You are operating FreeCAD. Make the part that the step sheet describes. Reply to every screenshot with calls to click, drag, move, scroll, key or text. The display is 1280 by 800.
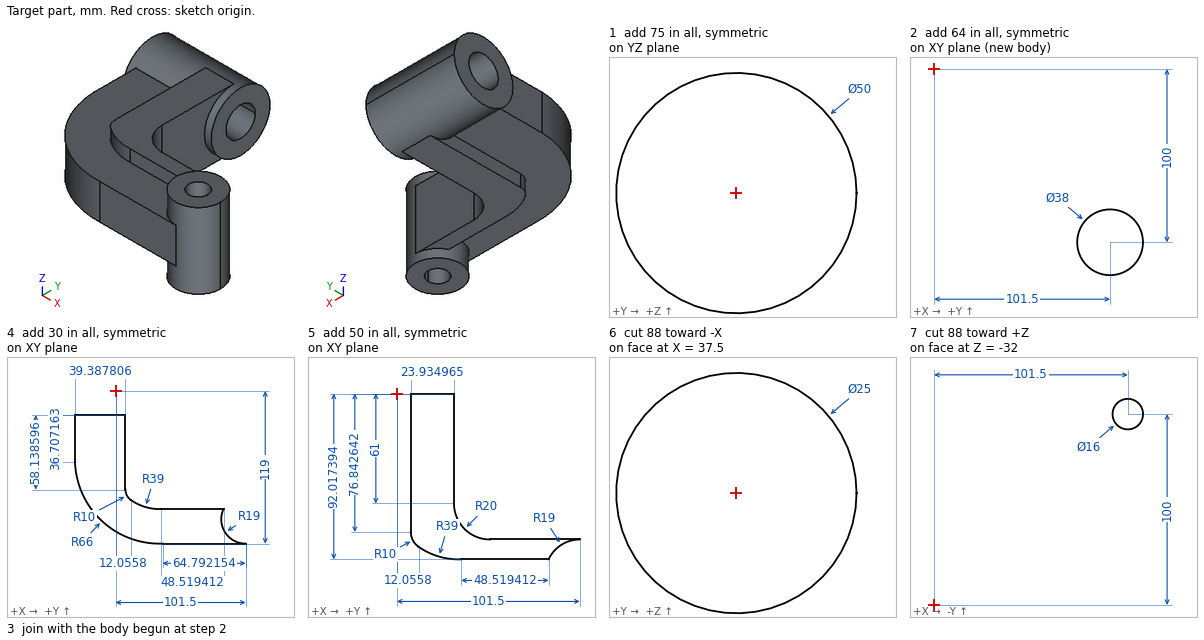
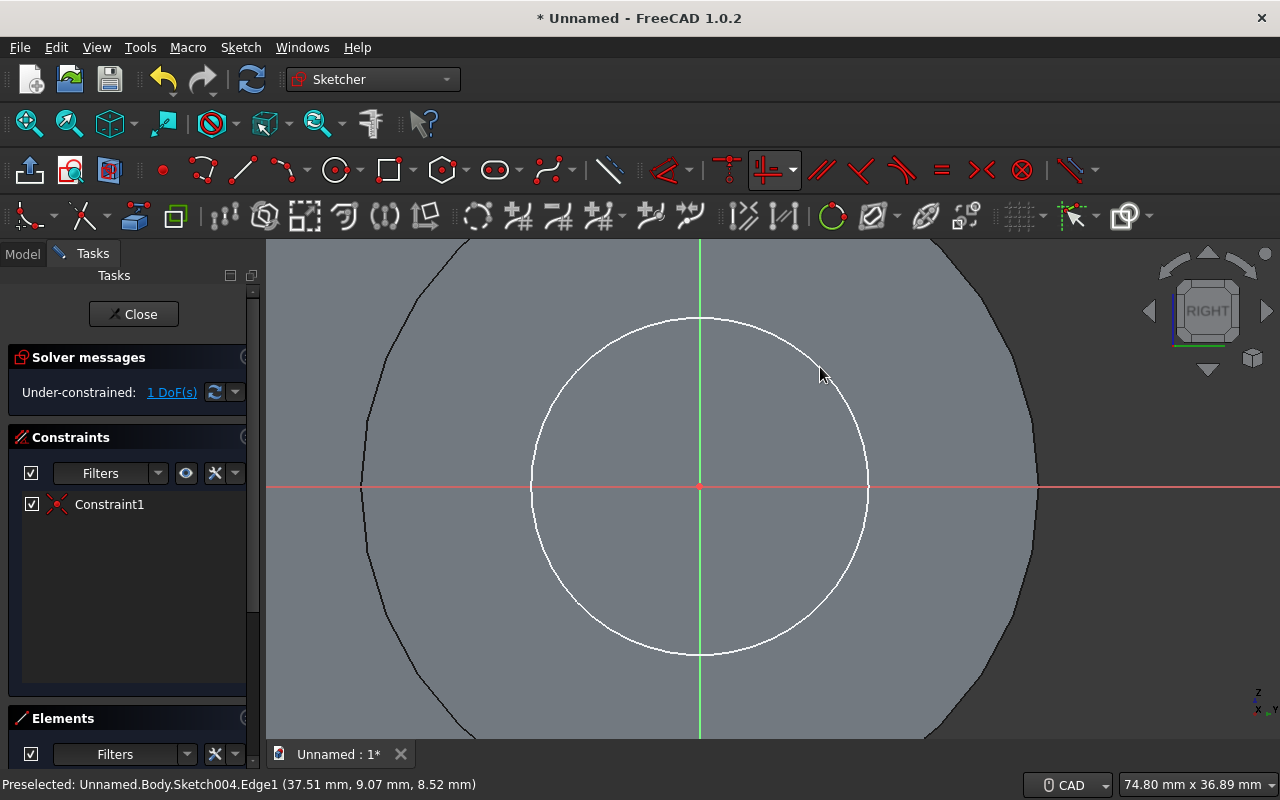
key(d)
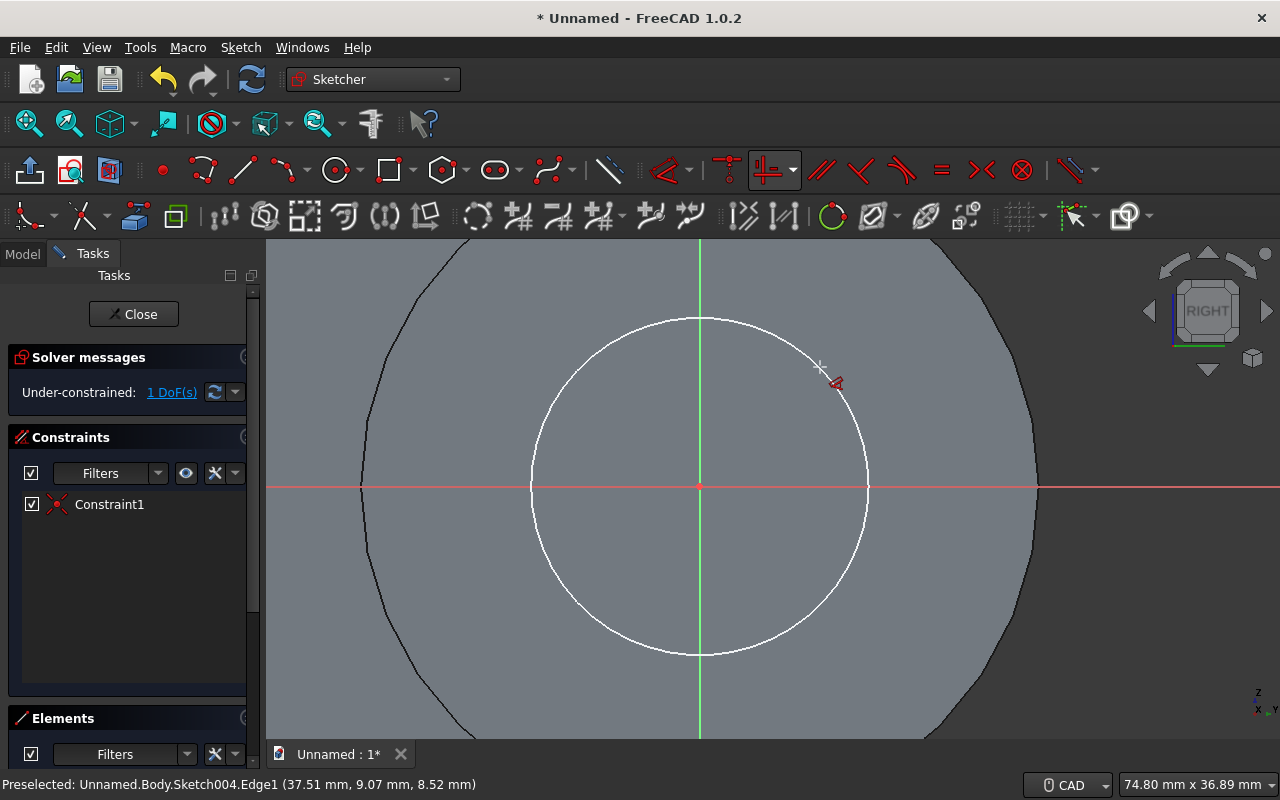
click(819, 367)
click(842, 344)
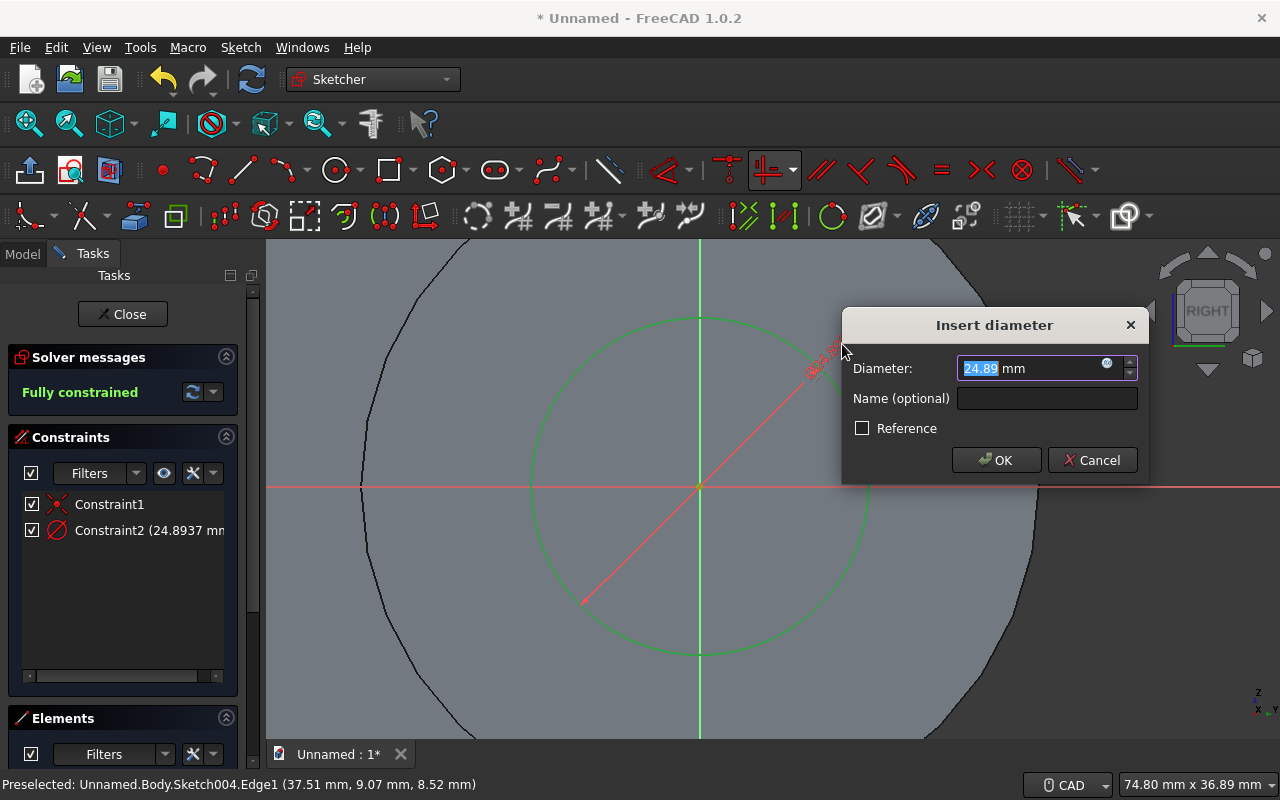
text(25)
key(Return)
key(Escape)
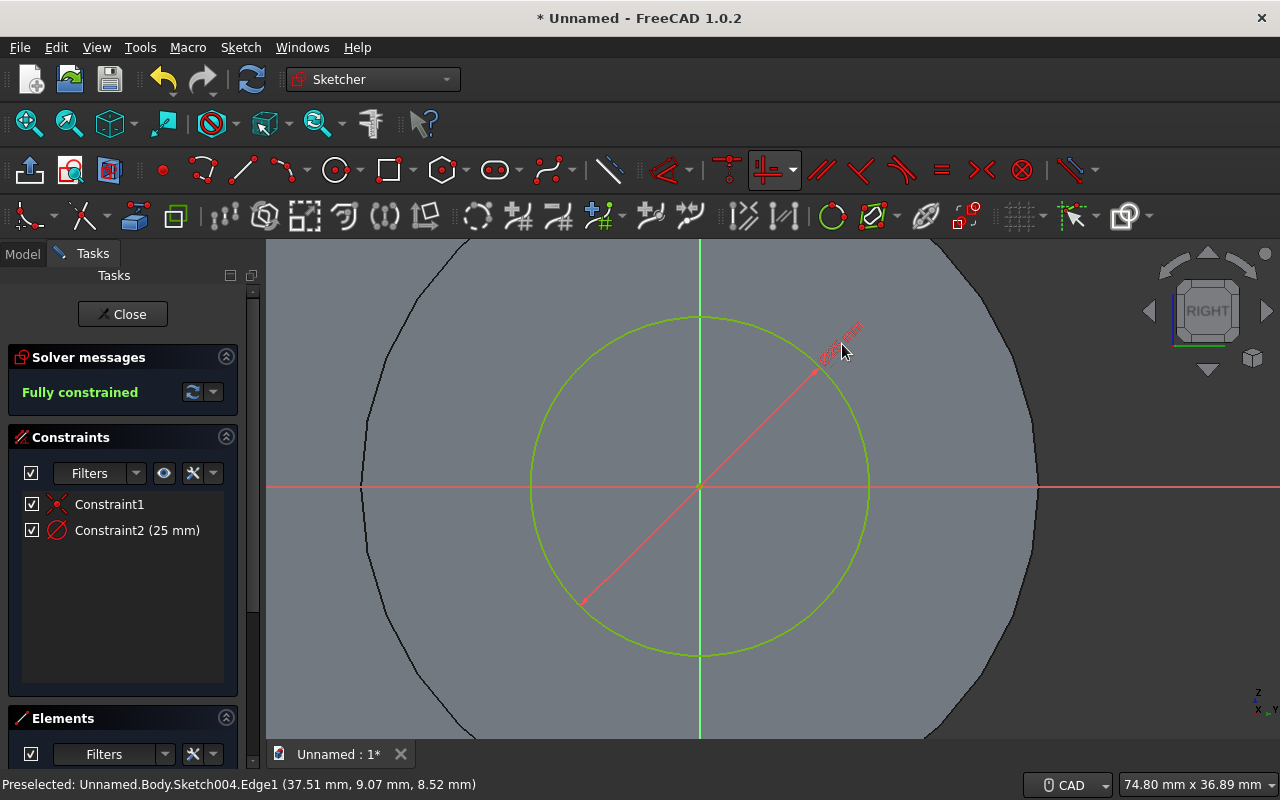
click(123, 314)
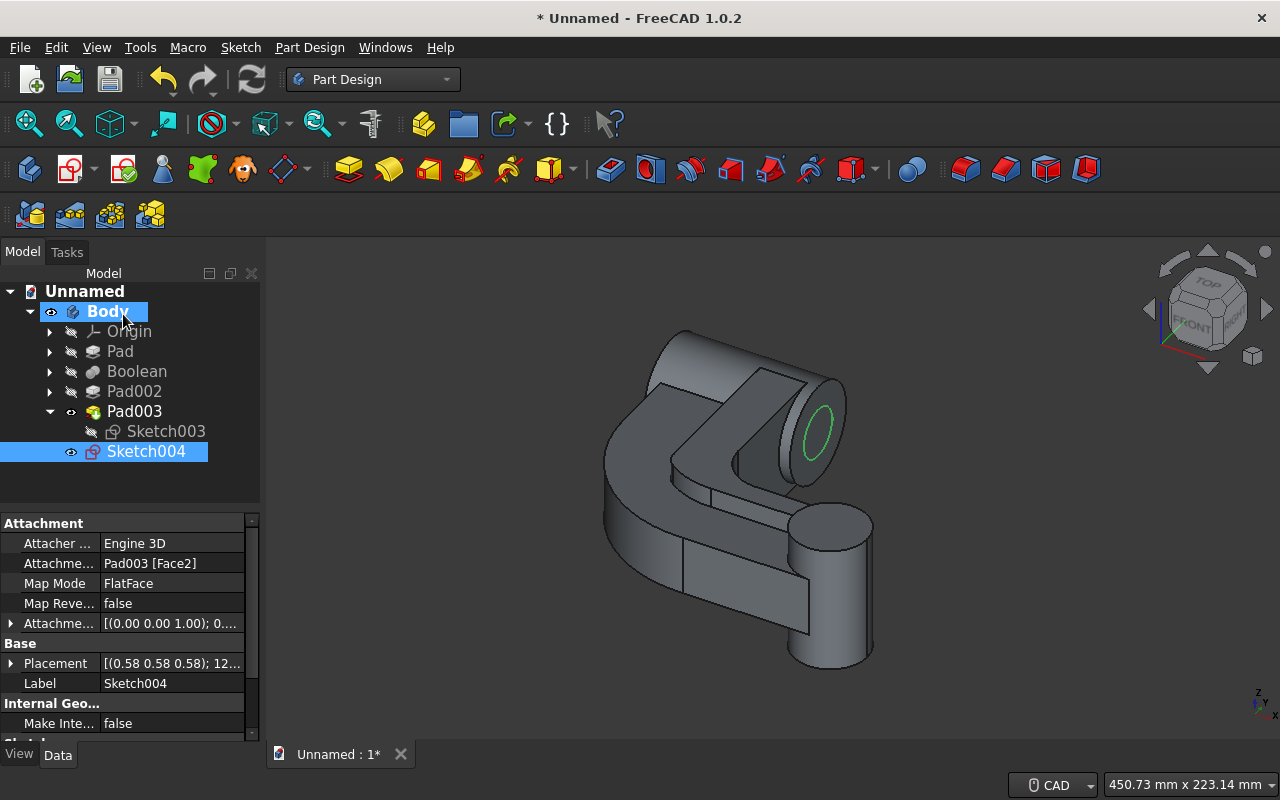
click(612, 170)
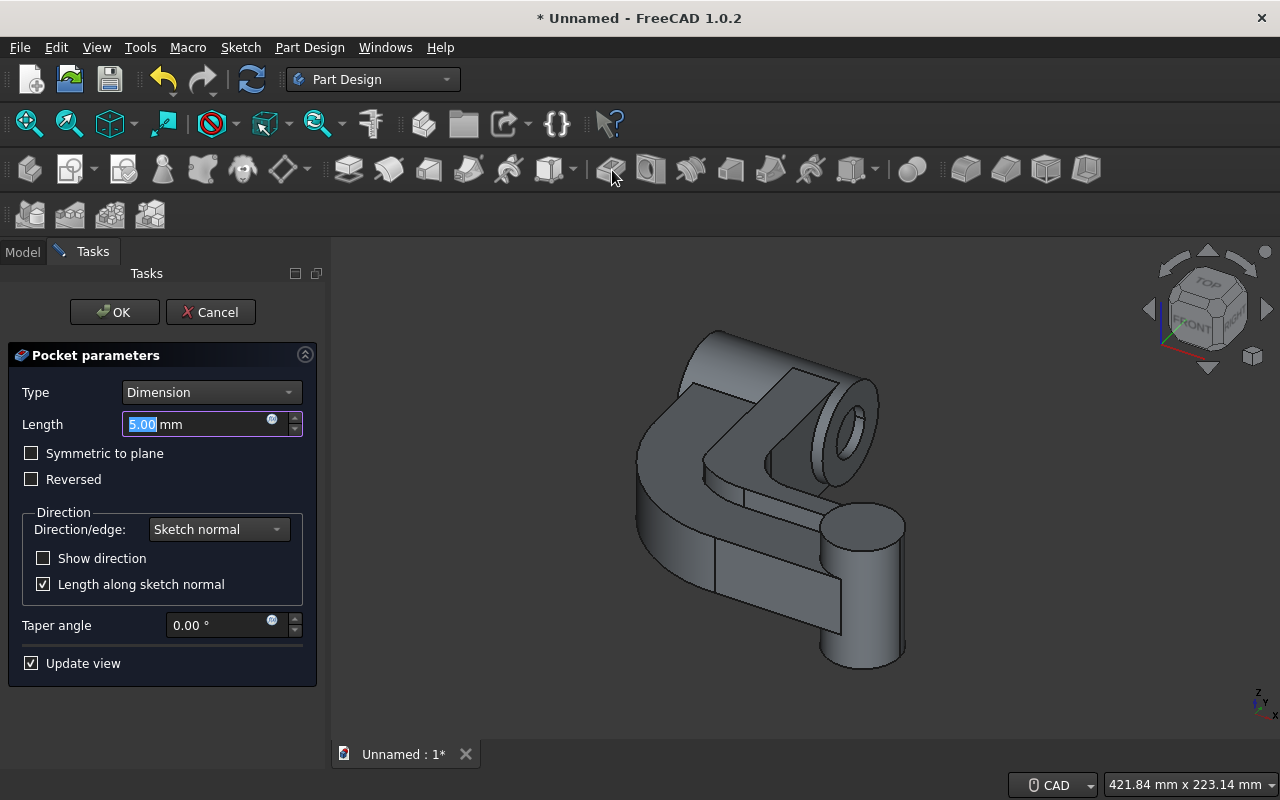
text(88)
key(Tab)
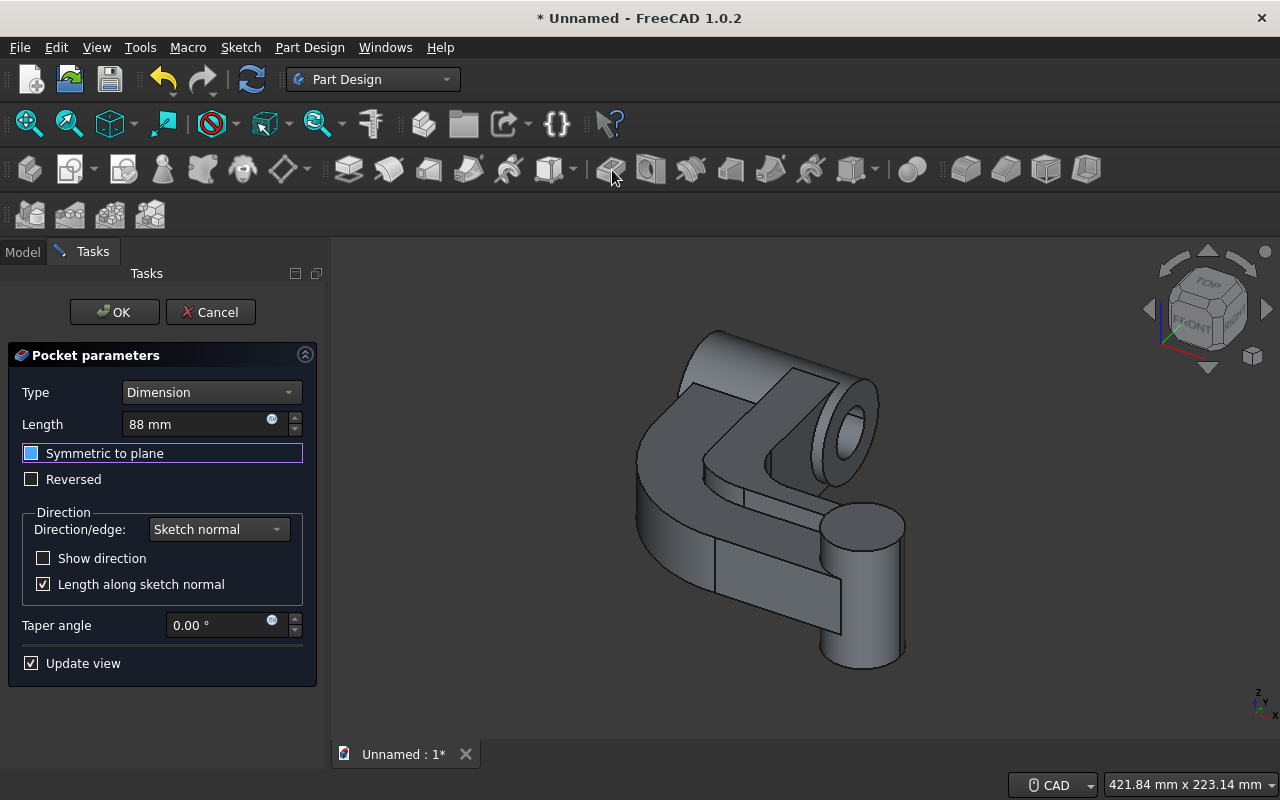
click(115, 312)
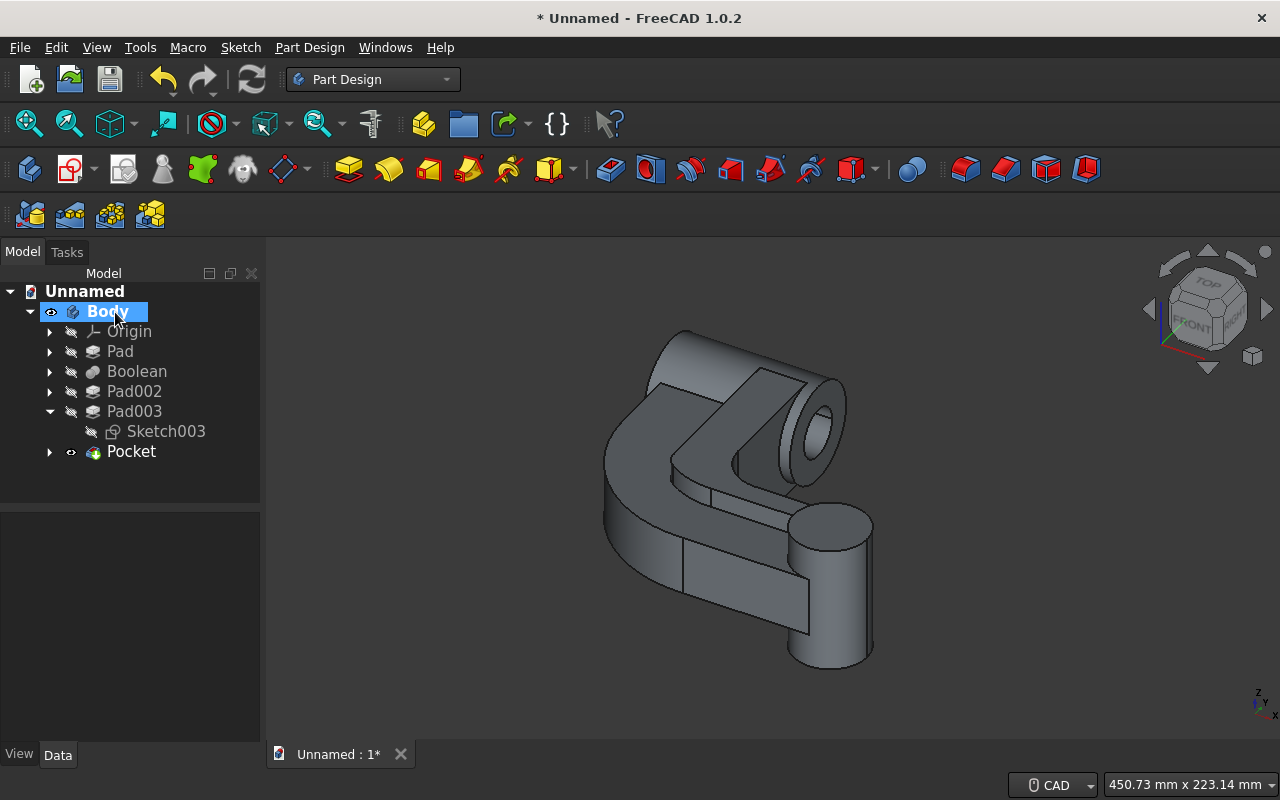
key(5)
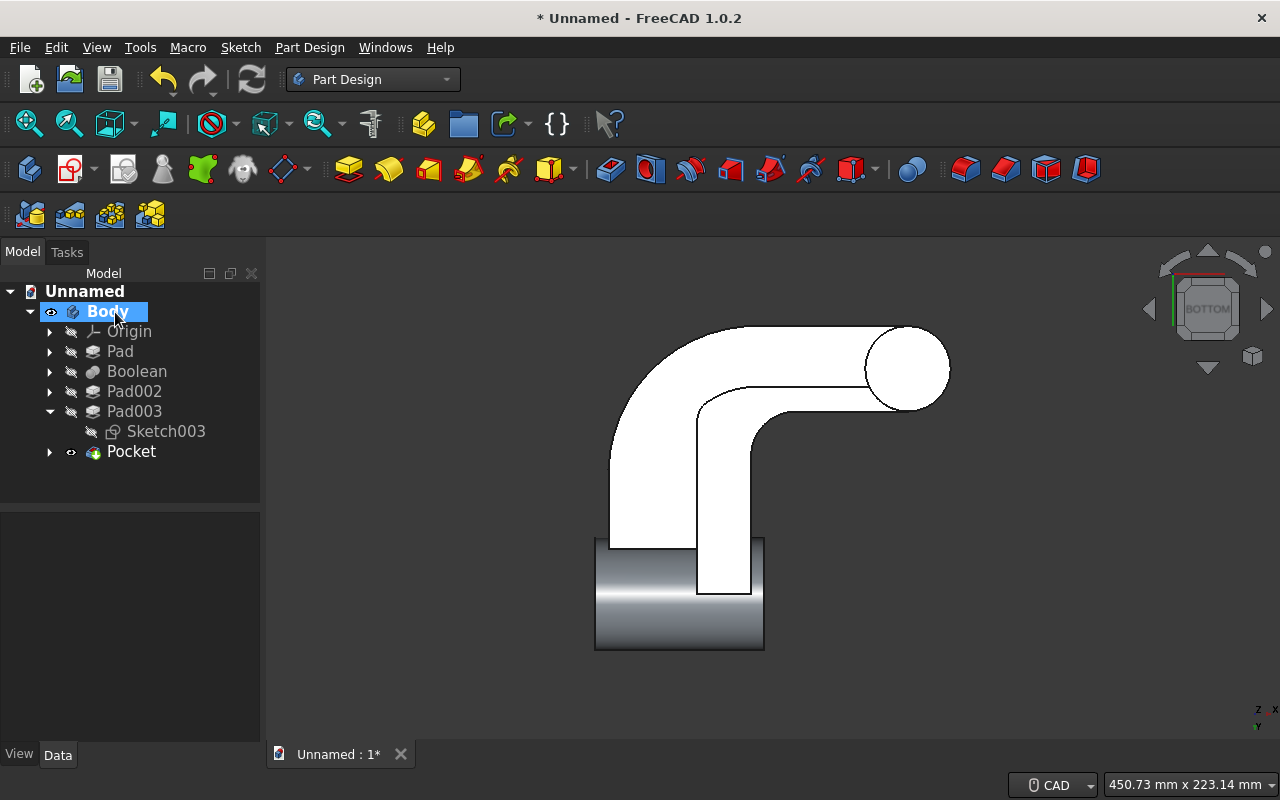
click(908, 368)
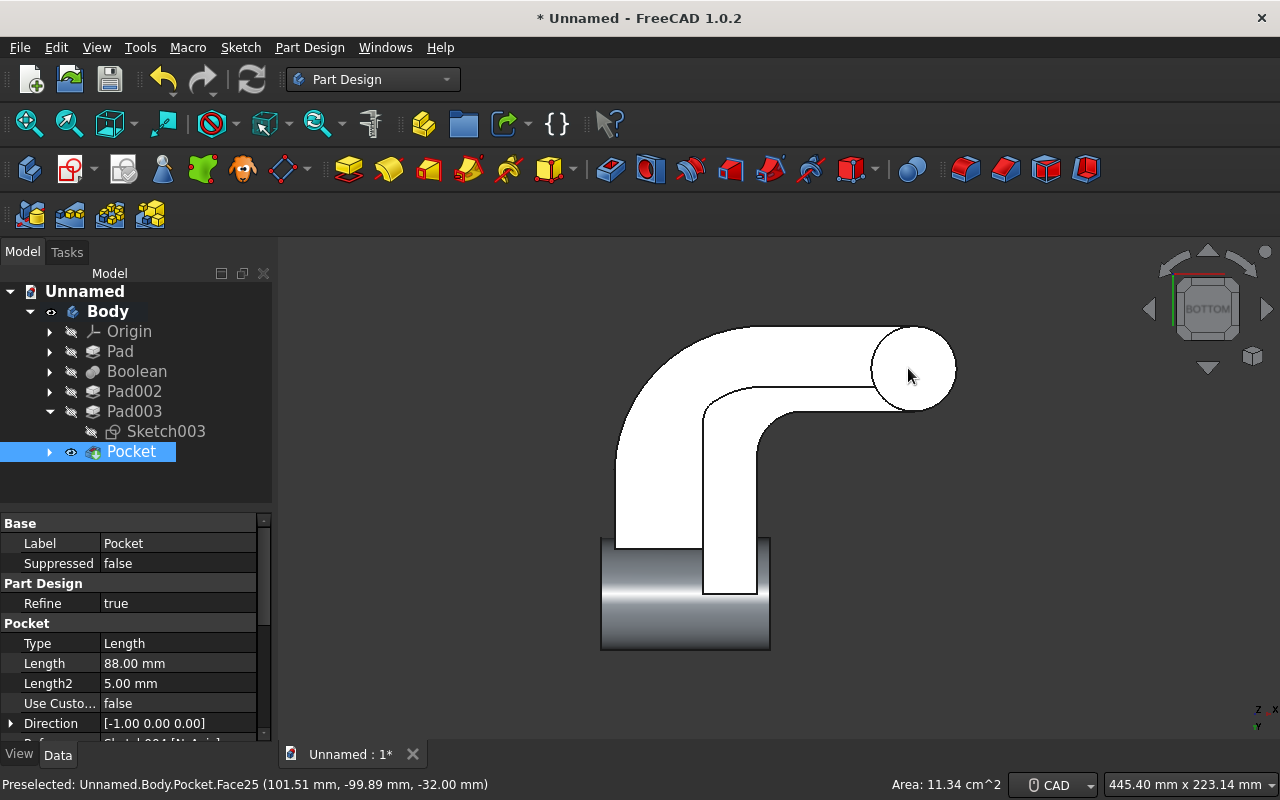
click(70, 170)